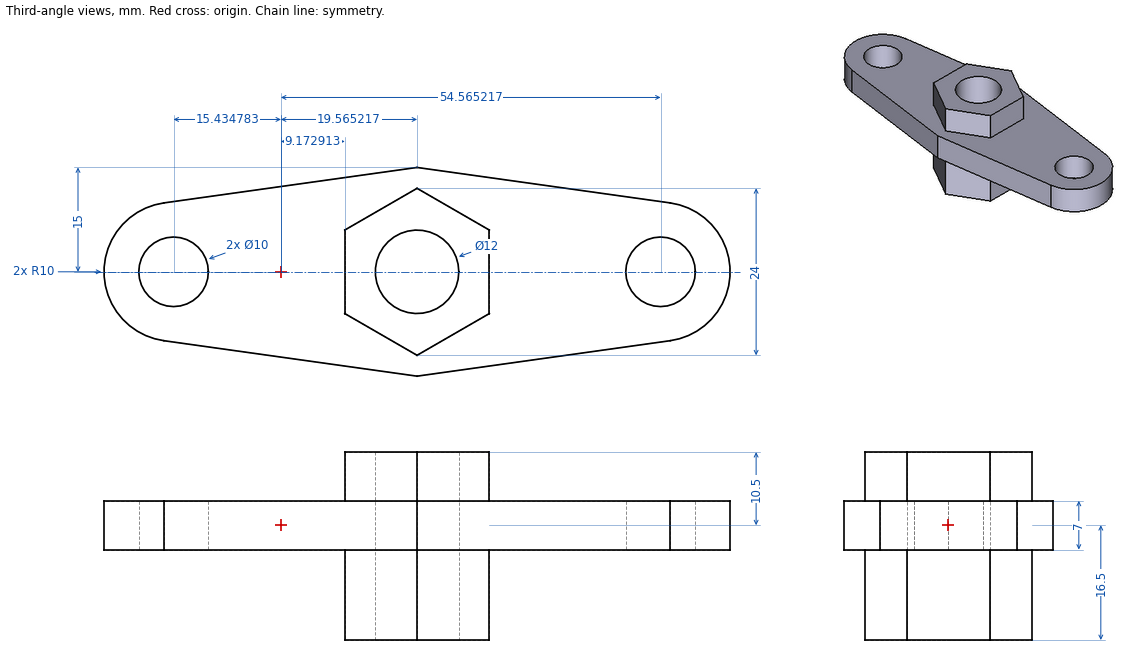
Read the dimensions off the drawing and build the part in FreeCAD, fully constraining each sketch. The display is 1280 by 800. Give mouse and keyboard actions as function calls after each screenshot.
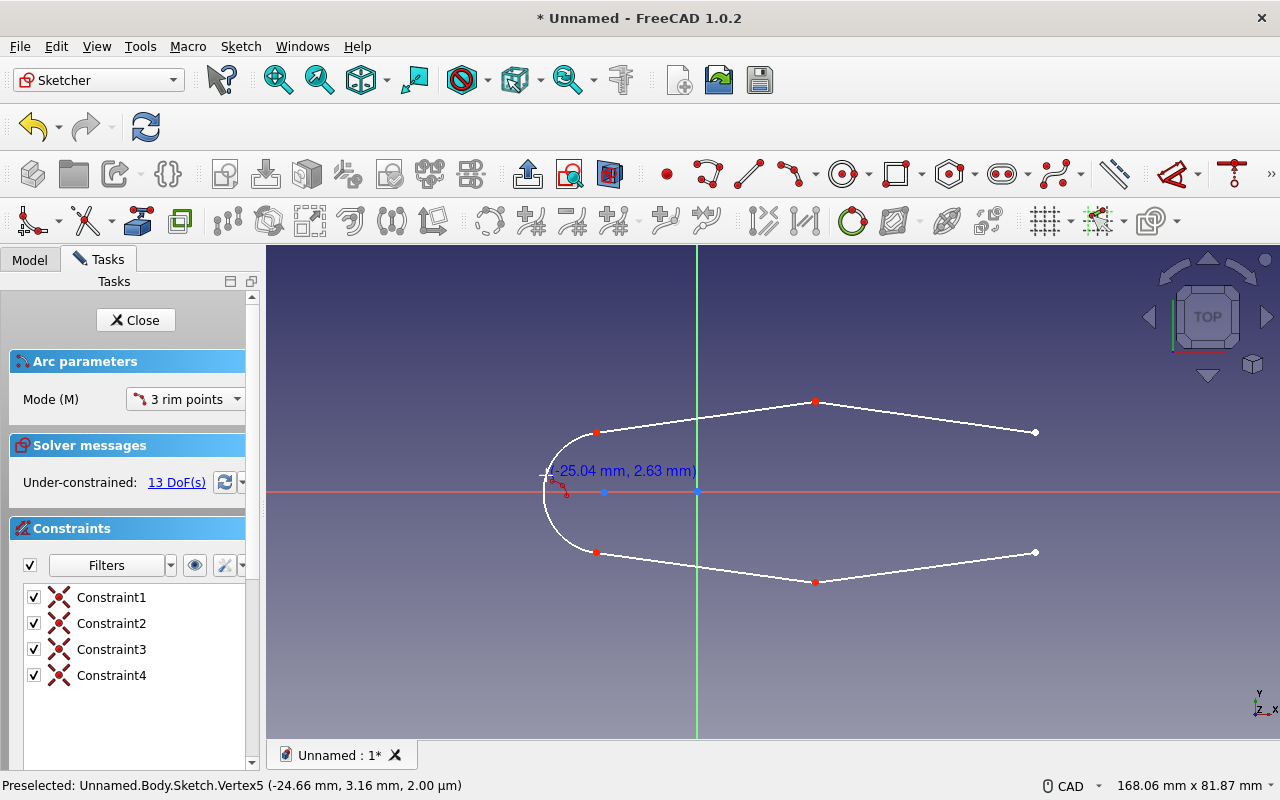
click(1035, 553)
click(1035, 433)
click(1084, 509)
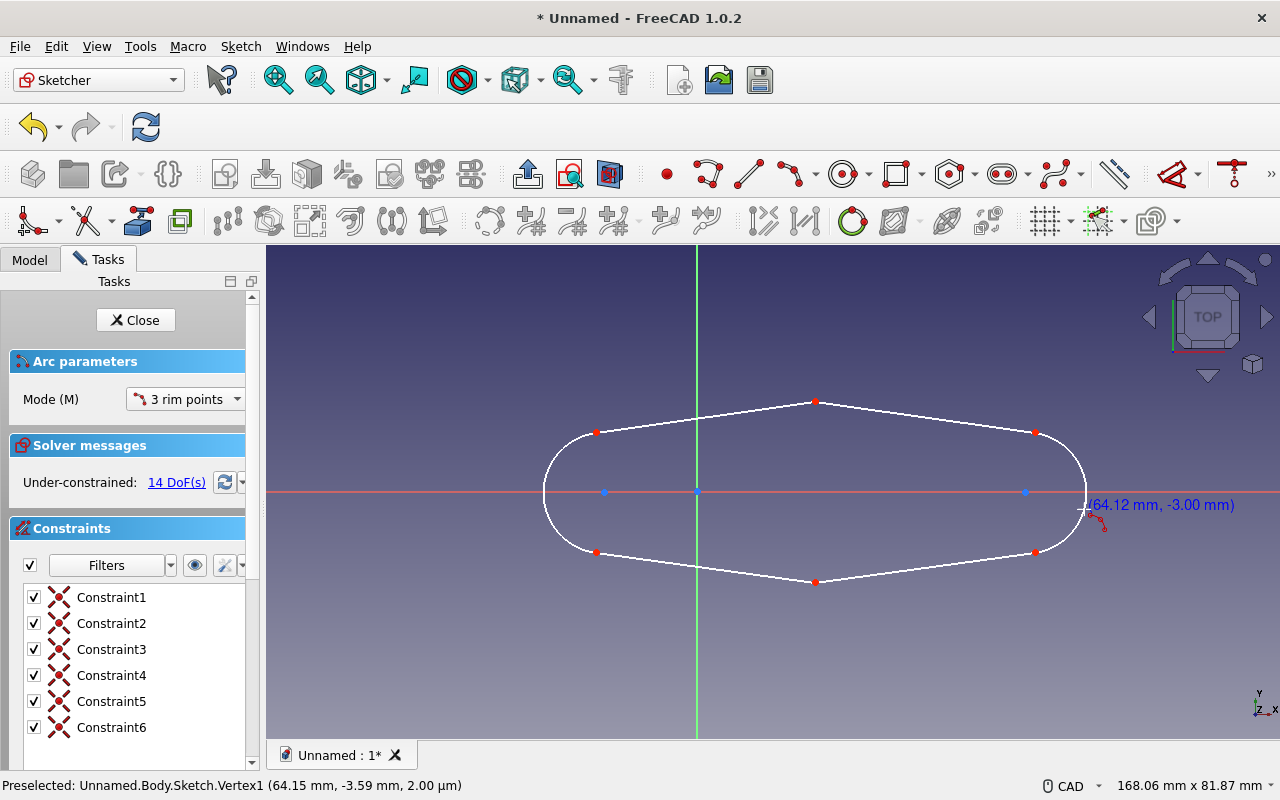
click(948, 174)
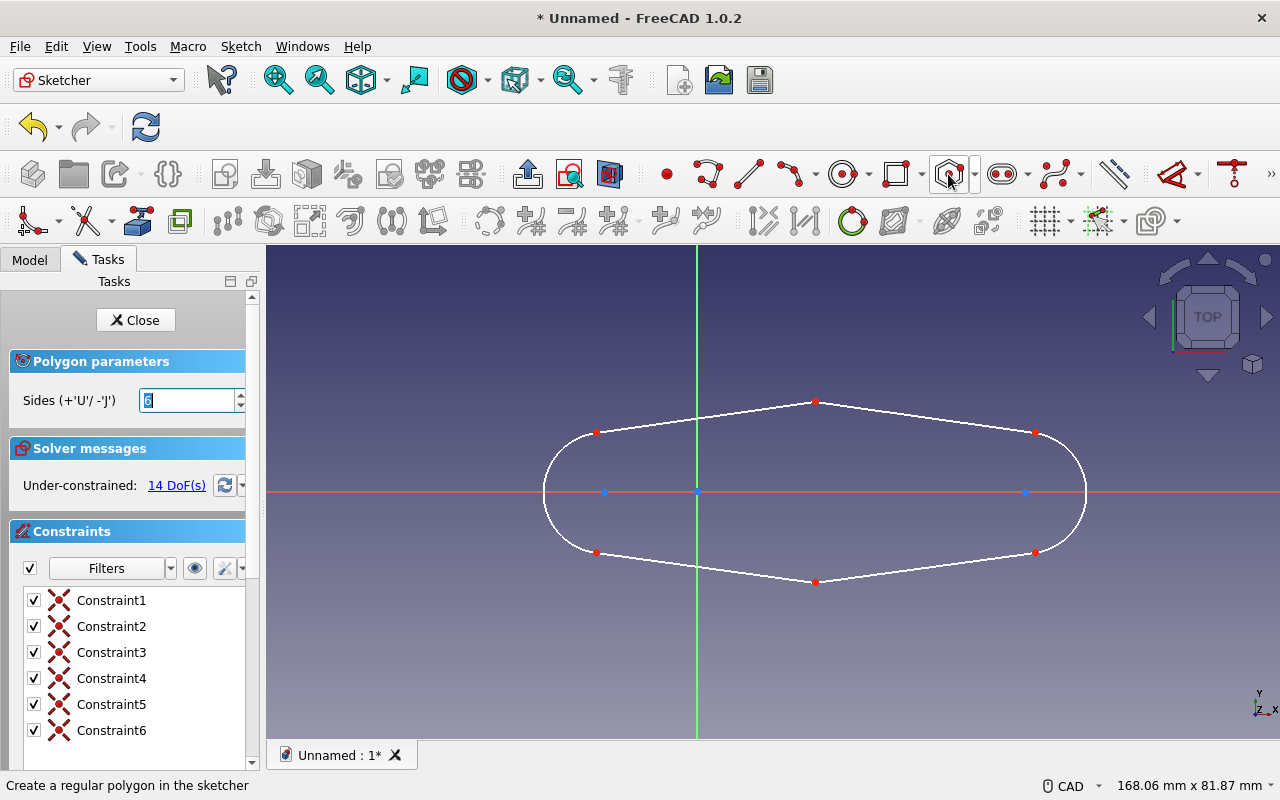
click(815, 492)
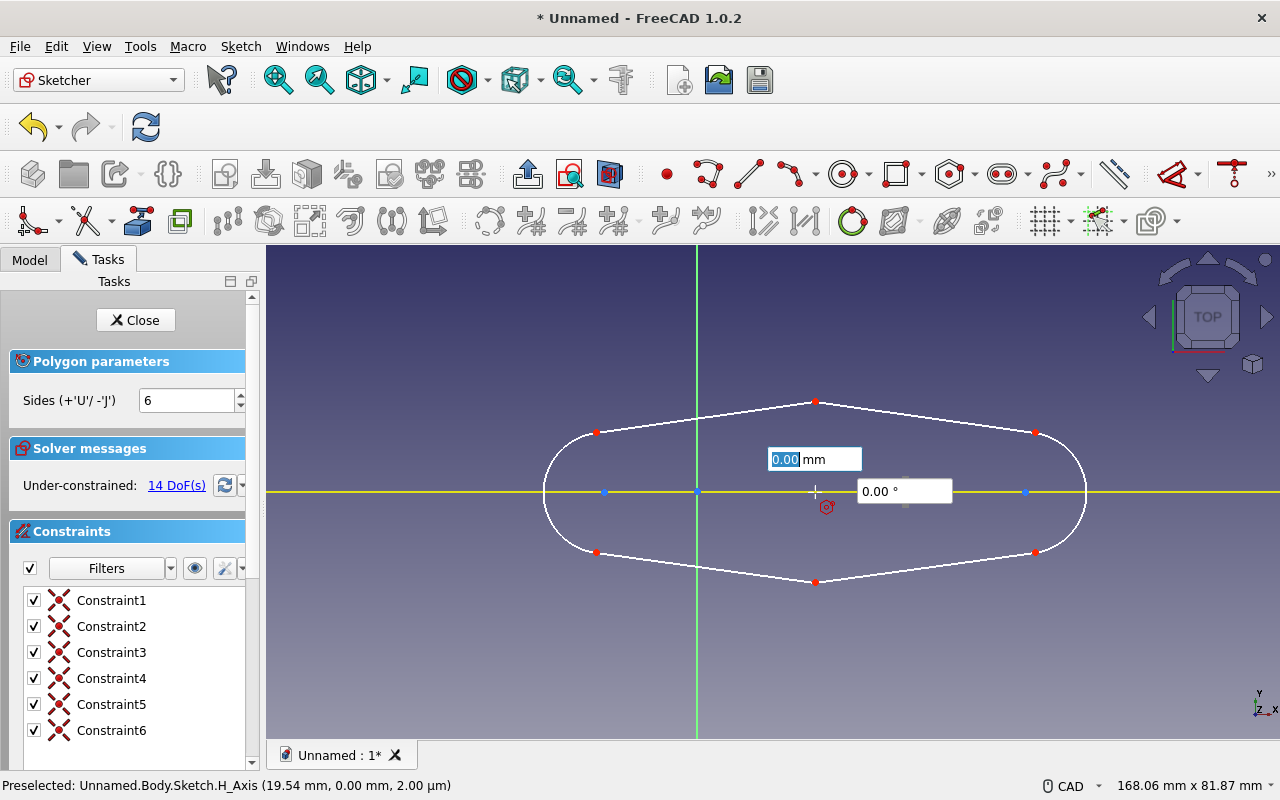
click(815, 419)
right_click(815, 419)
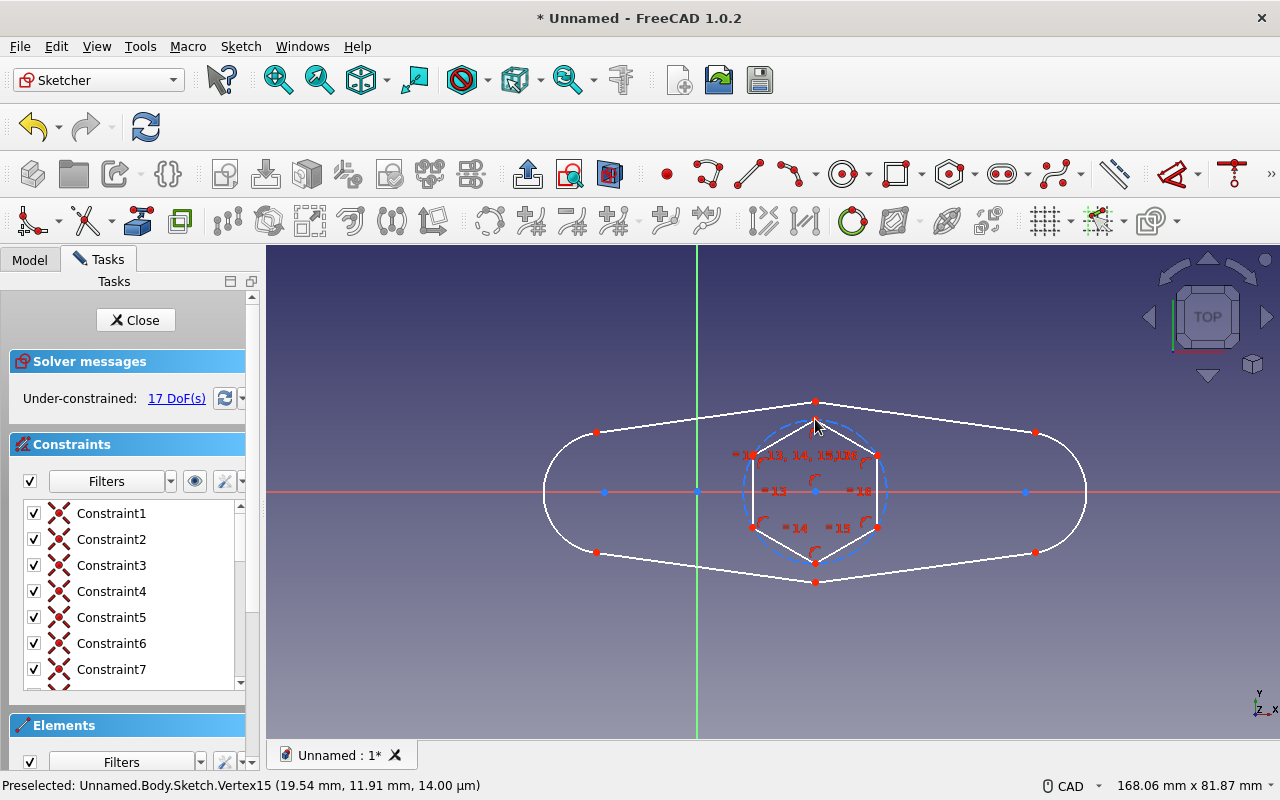
click(842, 174)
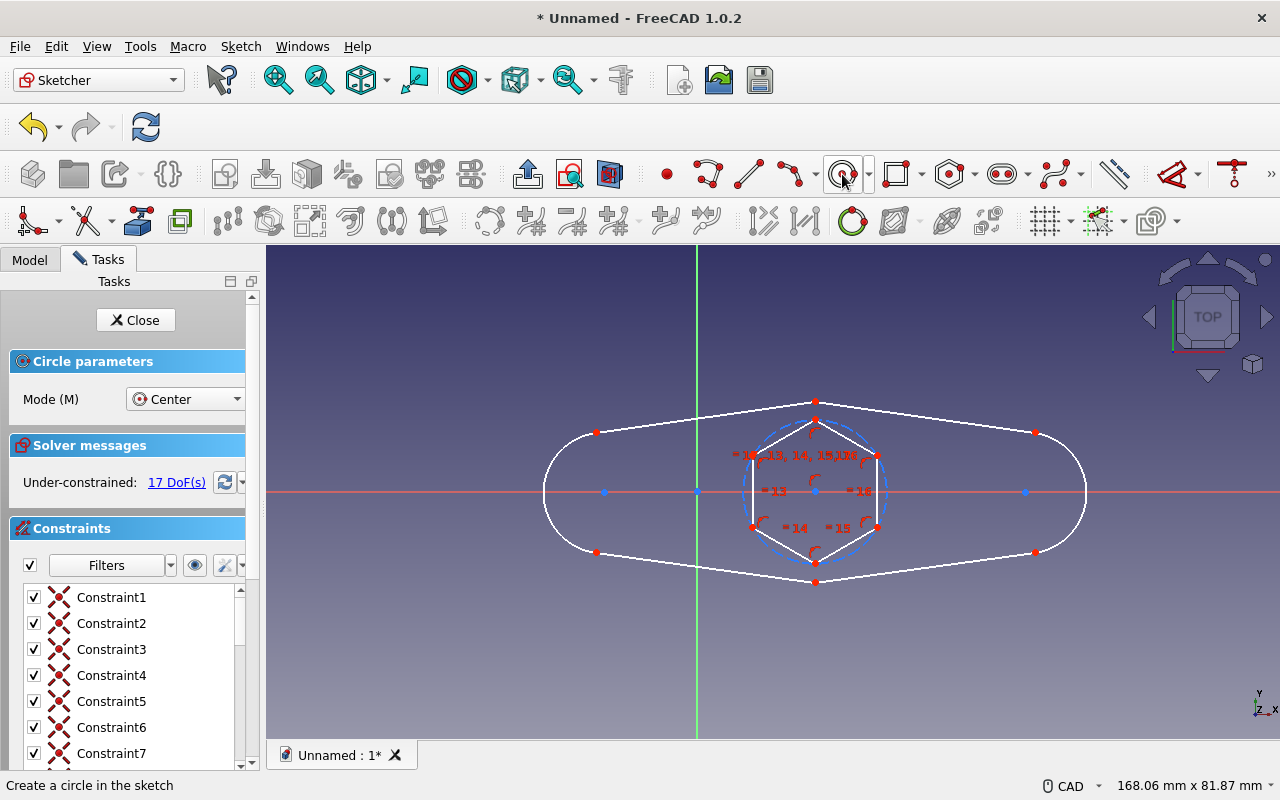
click(604, 492)
move(625, 471)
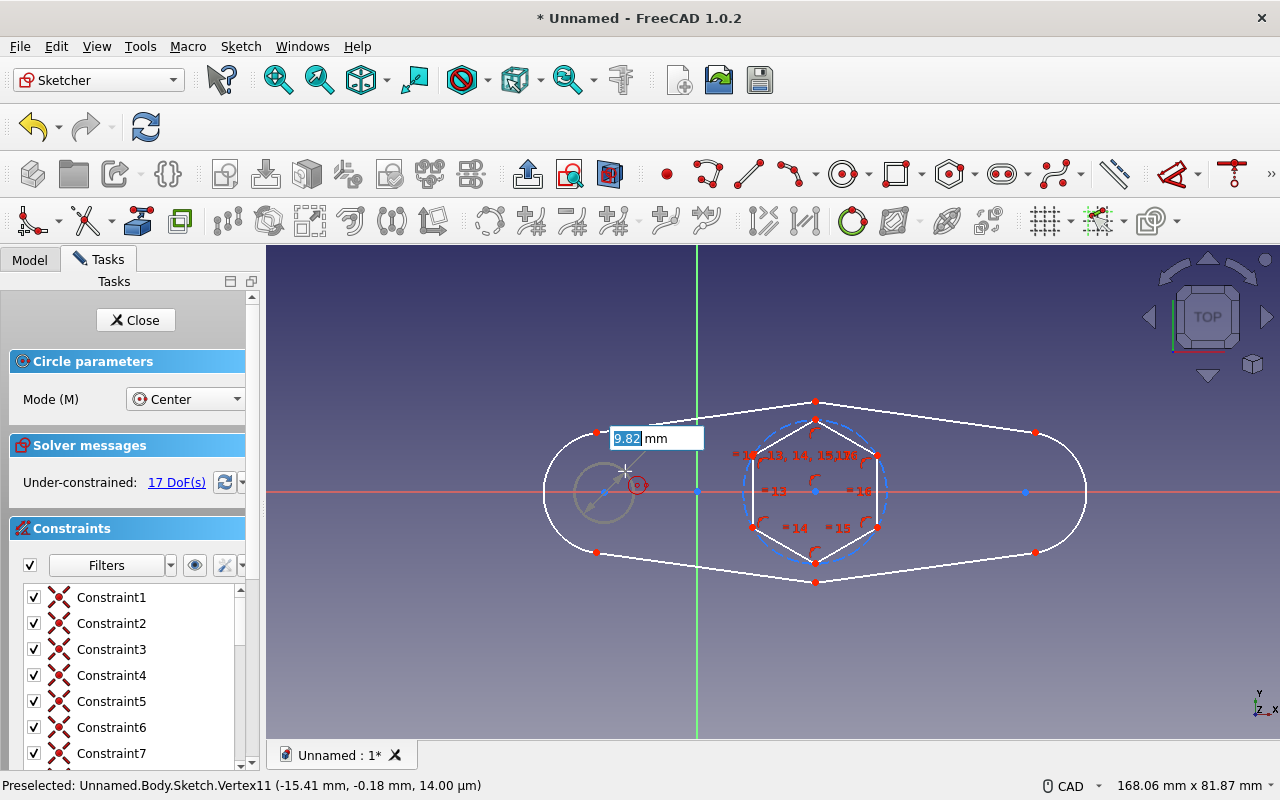
text(10)
key(Return)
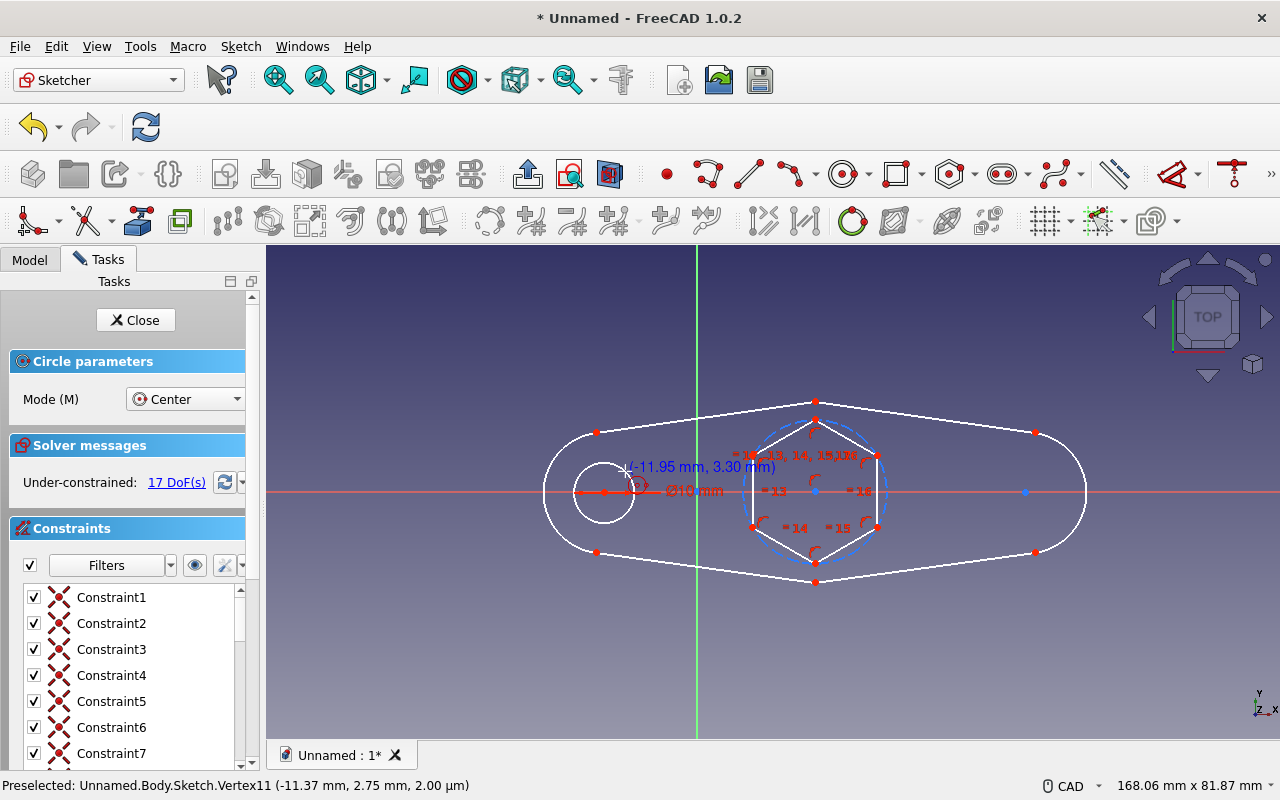
click(1026, 492)
move(1048, 471)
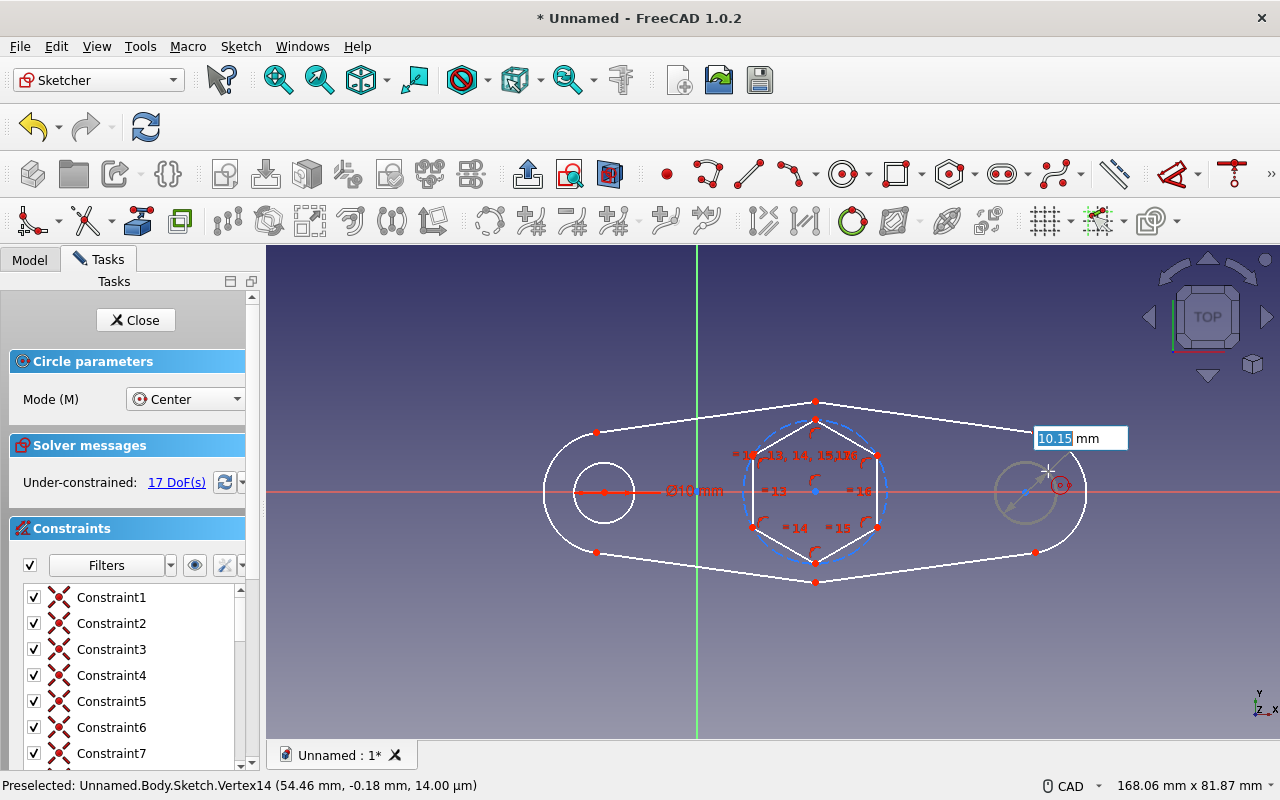
text(10)
key(Return)
key(Escape)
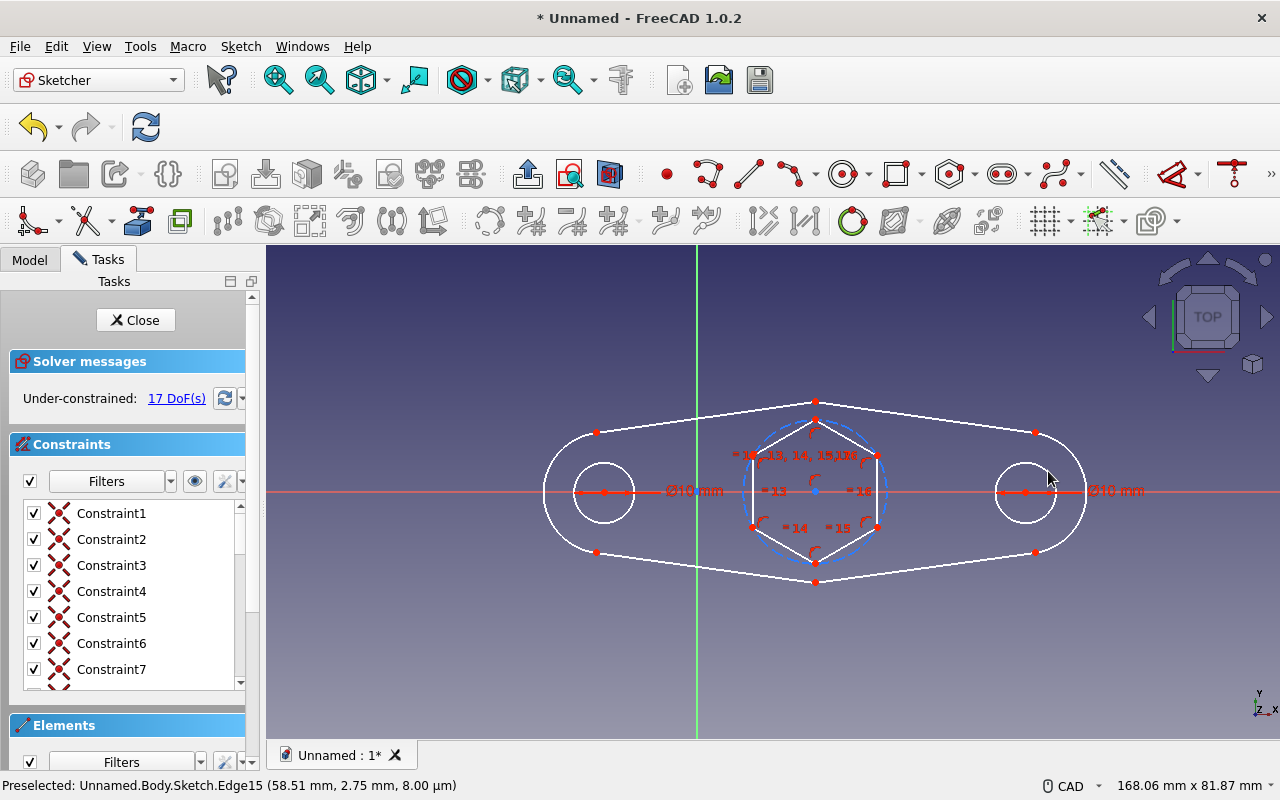
click(969, 424)